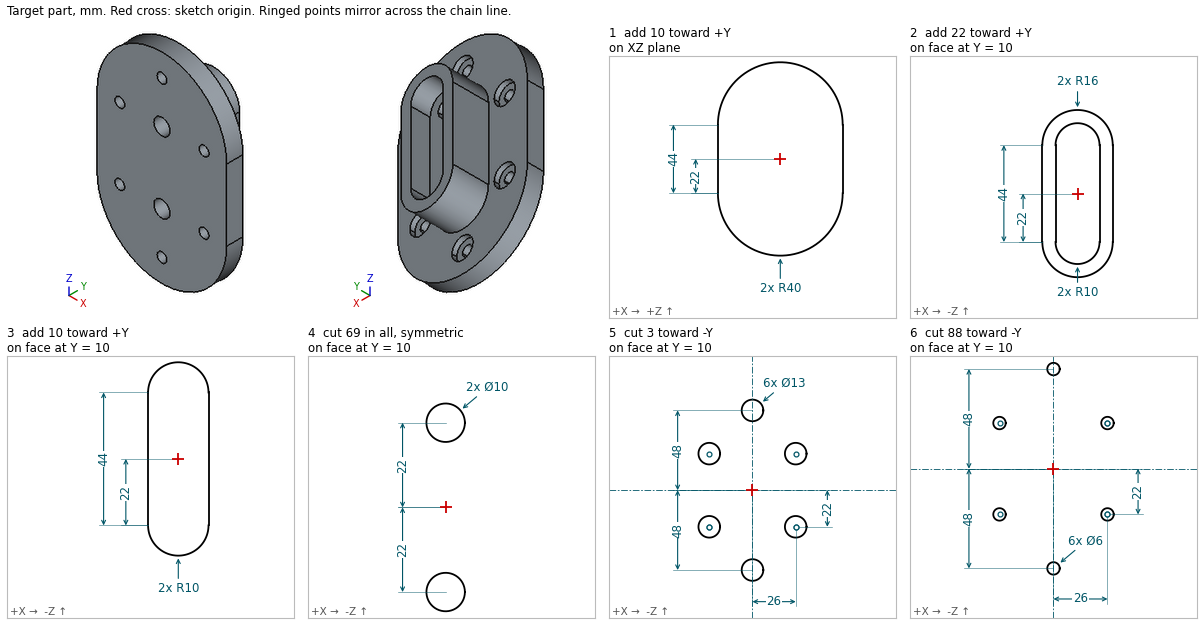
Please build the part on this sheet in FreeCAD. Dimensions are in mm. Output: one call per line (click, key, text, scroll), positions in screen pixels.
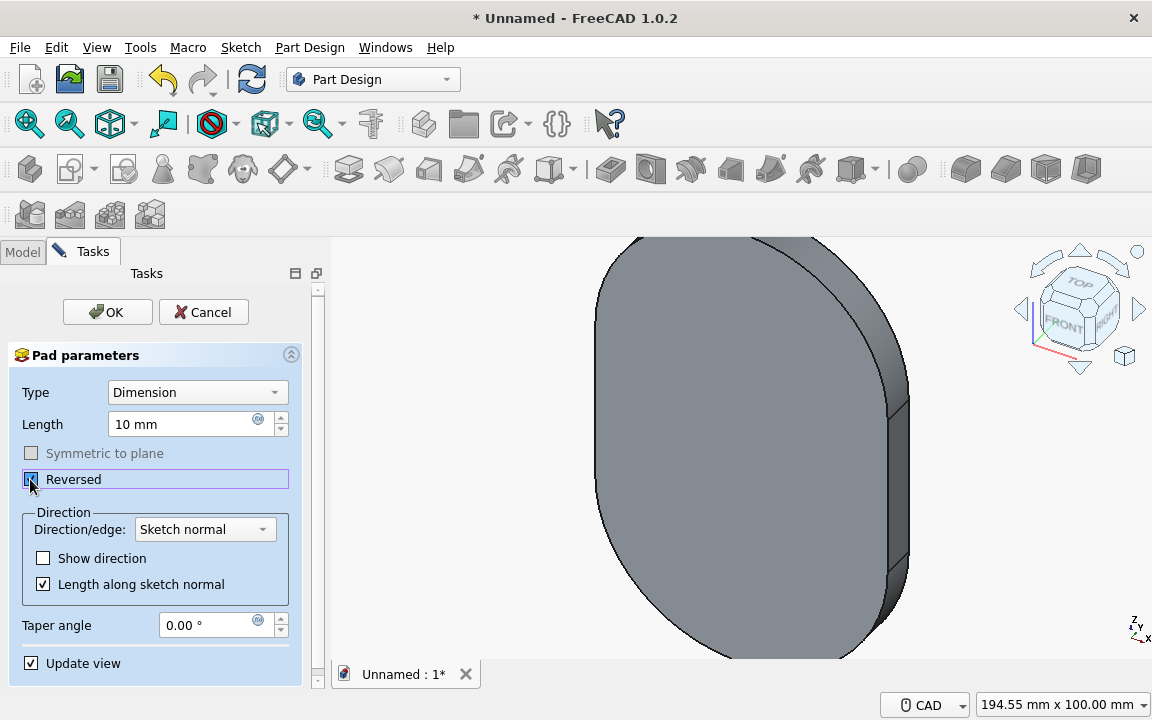
click(108, 312)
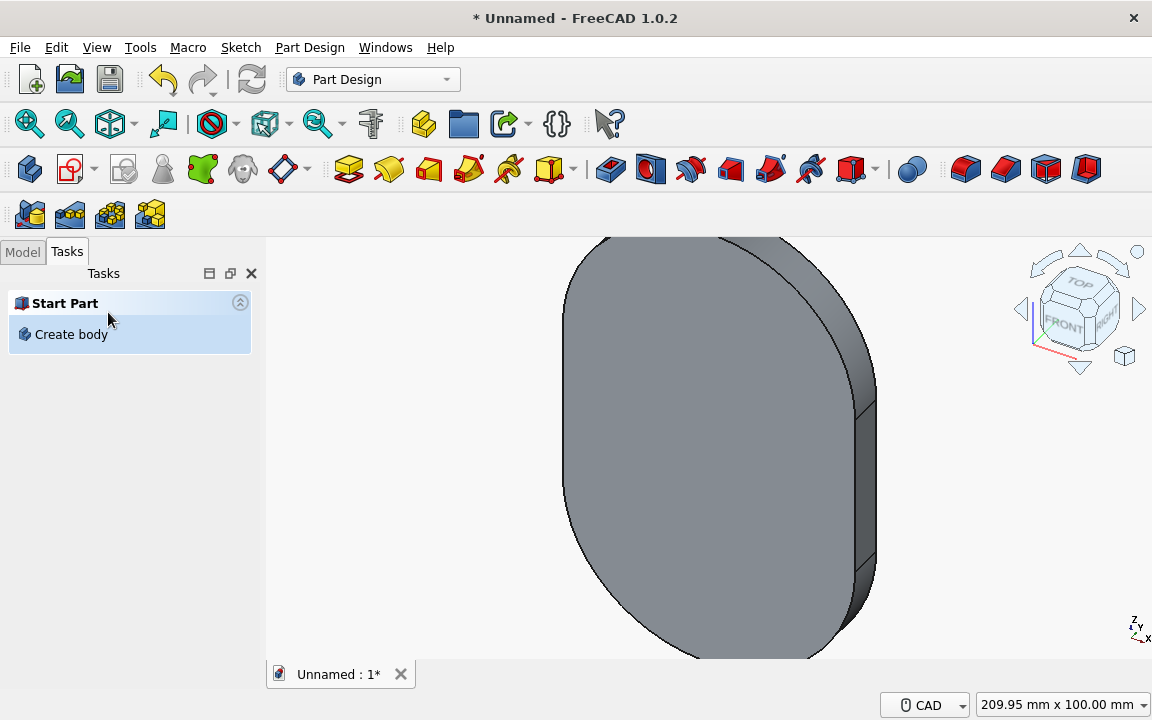
click(30, 124)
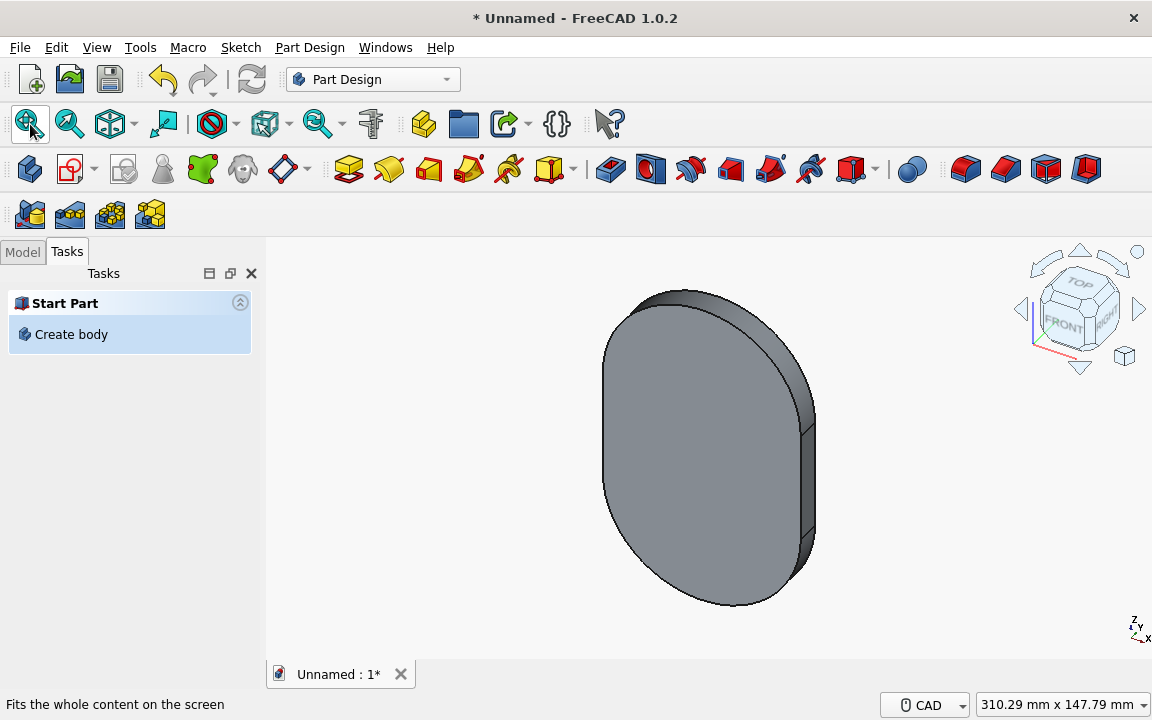
key(4)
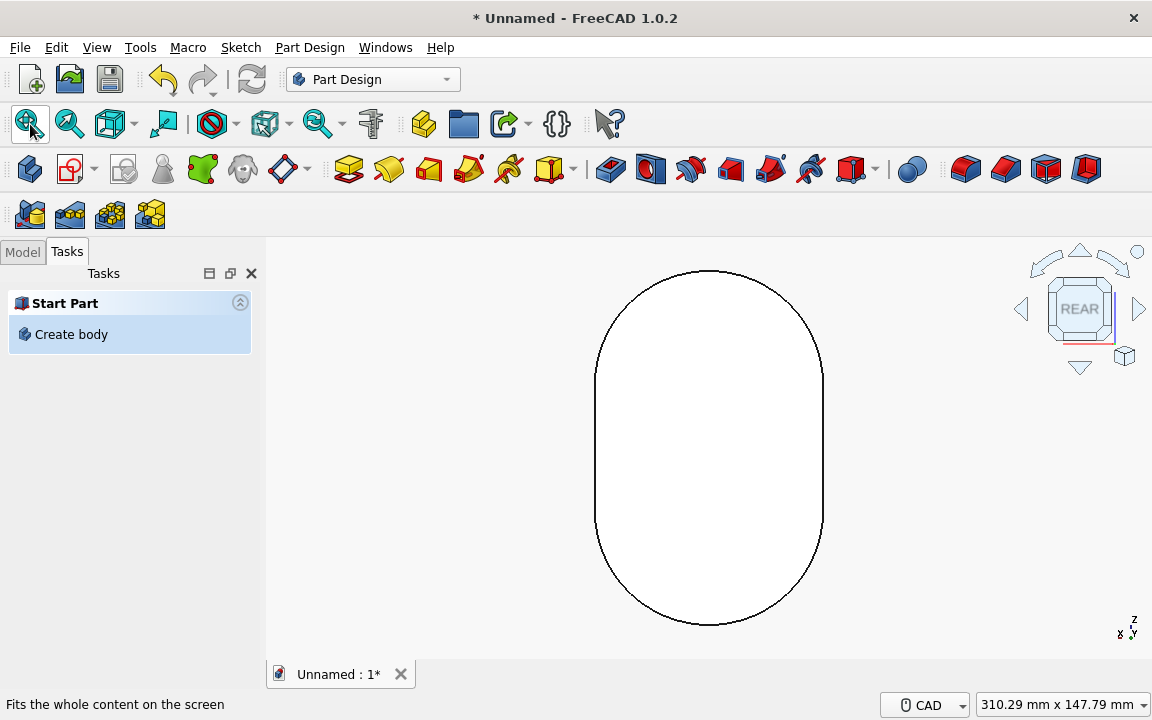
click(709, 396)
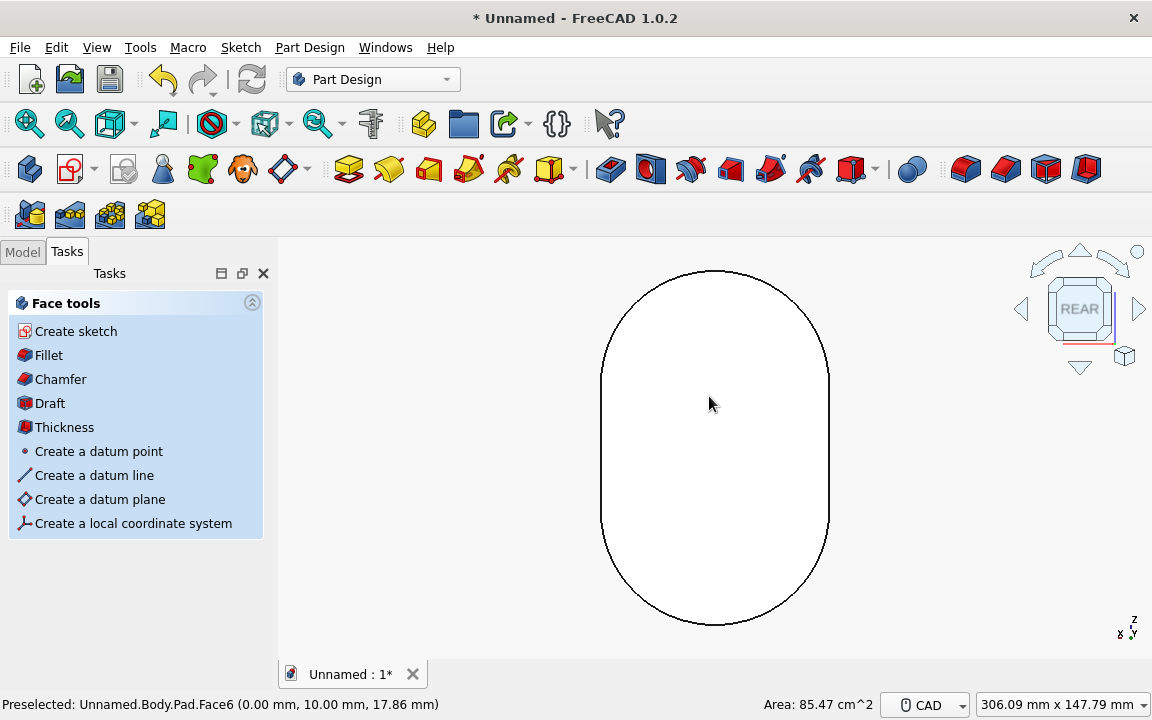
click(70, 170)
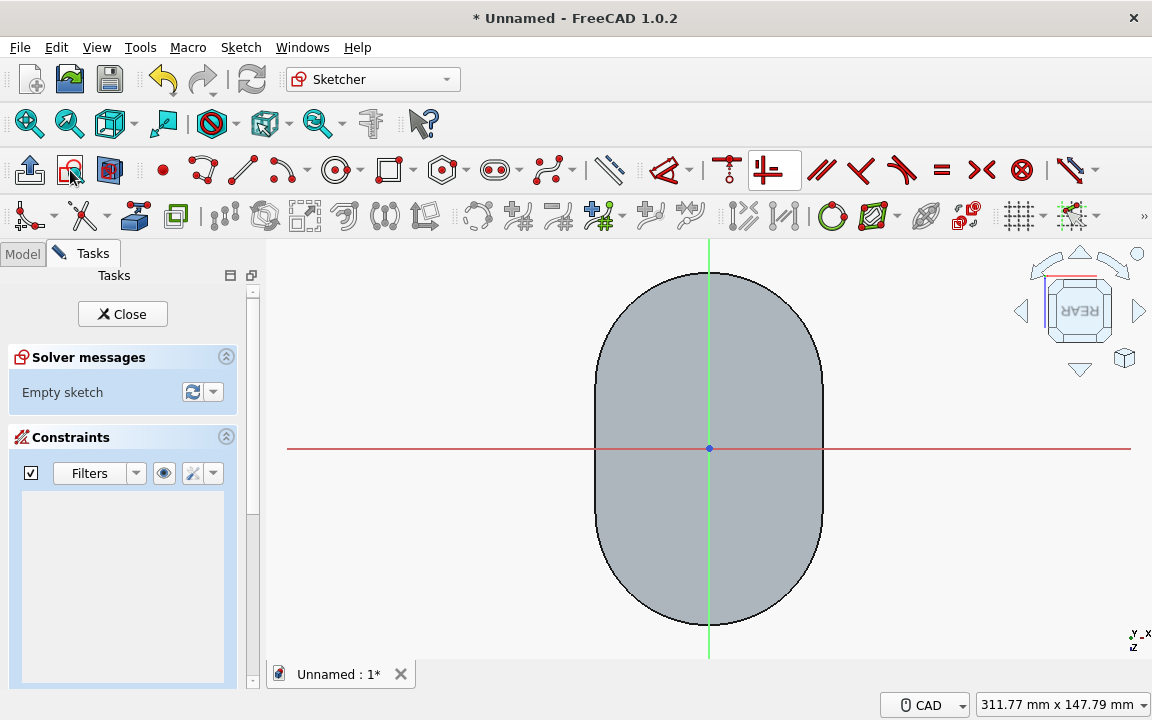
key(g)
key(s)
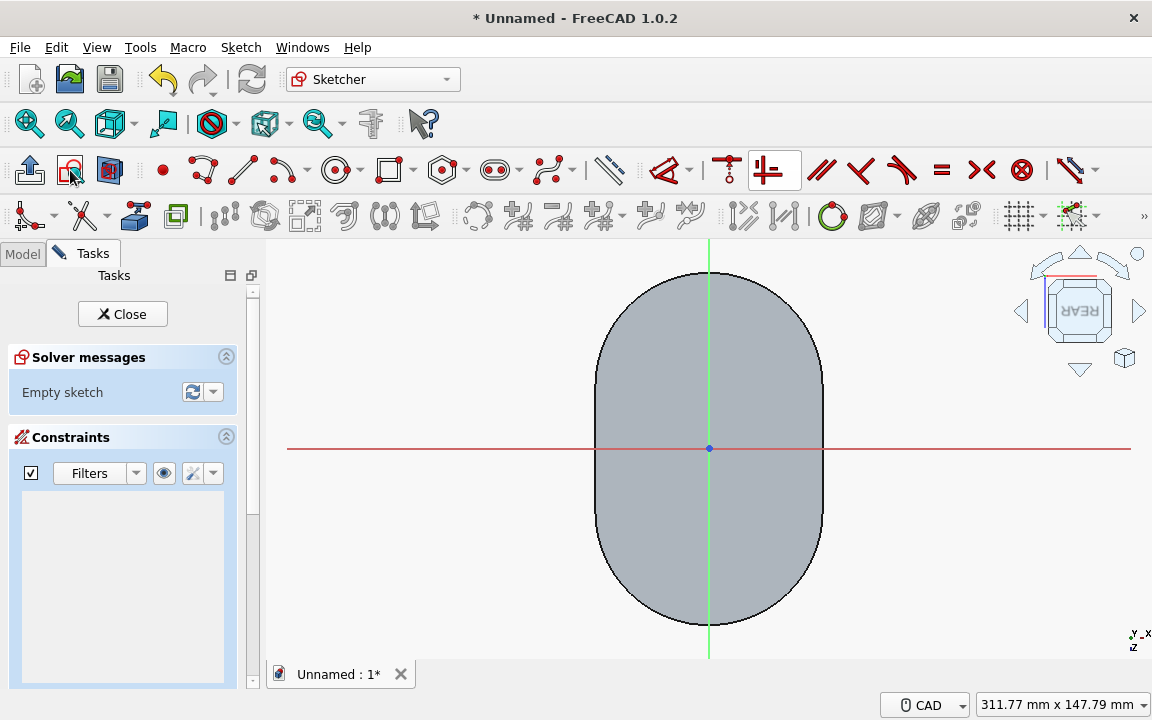
click(709, 512)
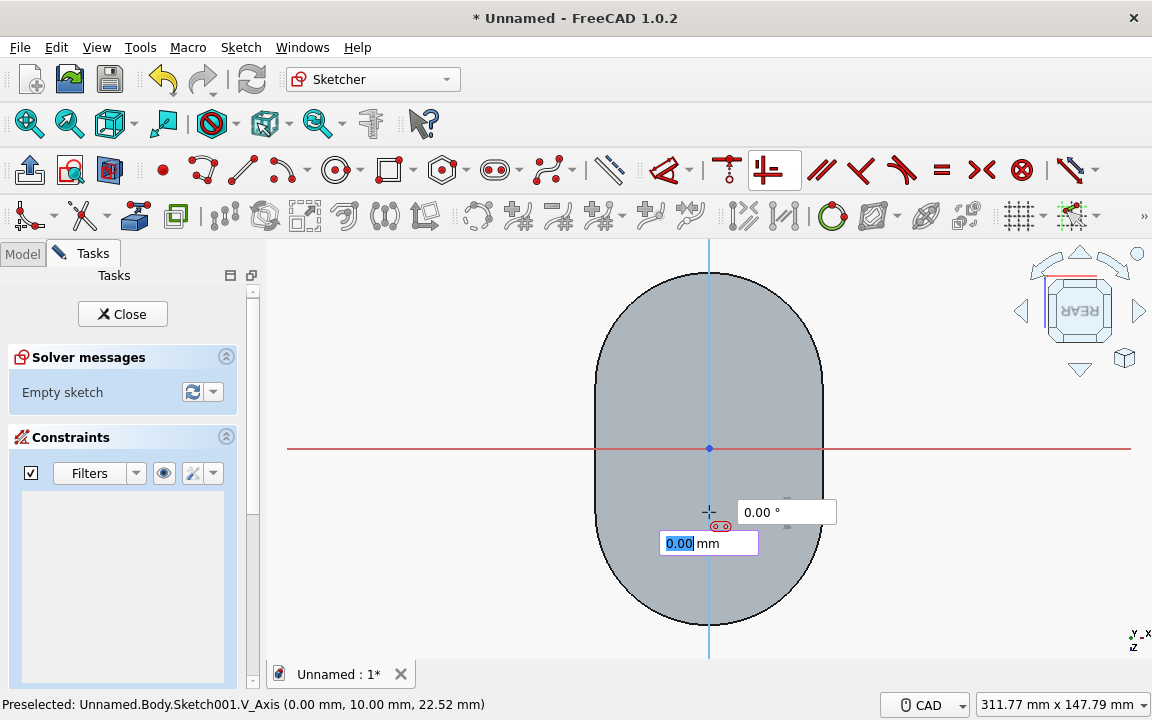
click(718, 386)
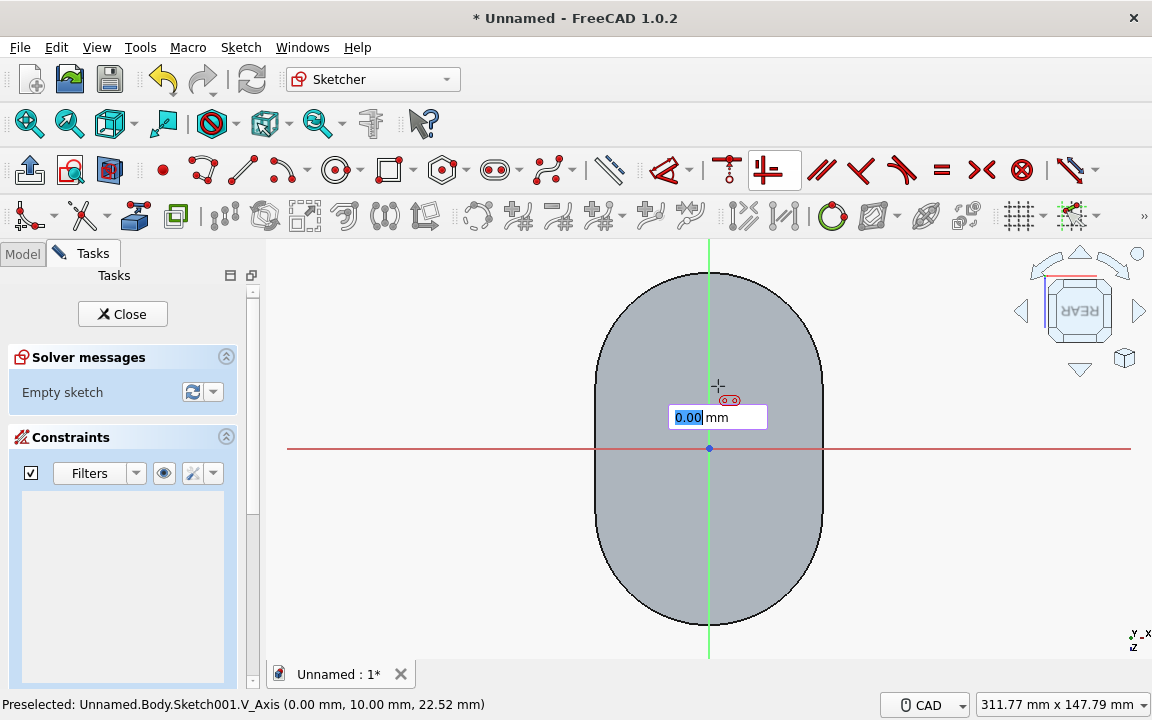
click(754, 468)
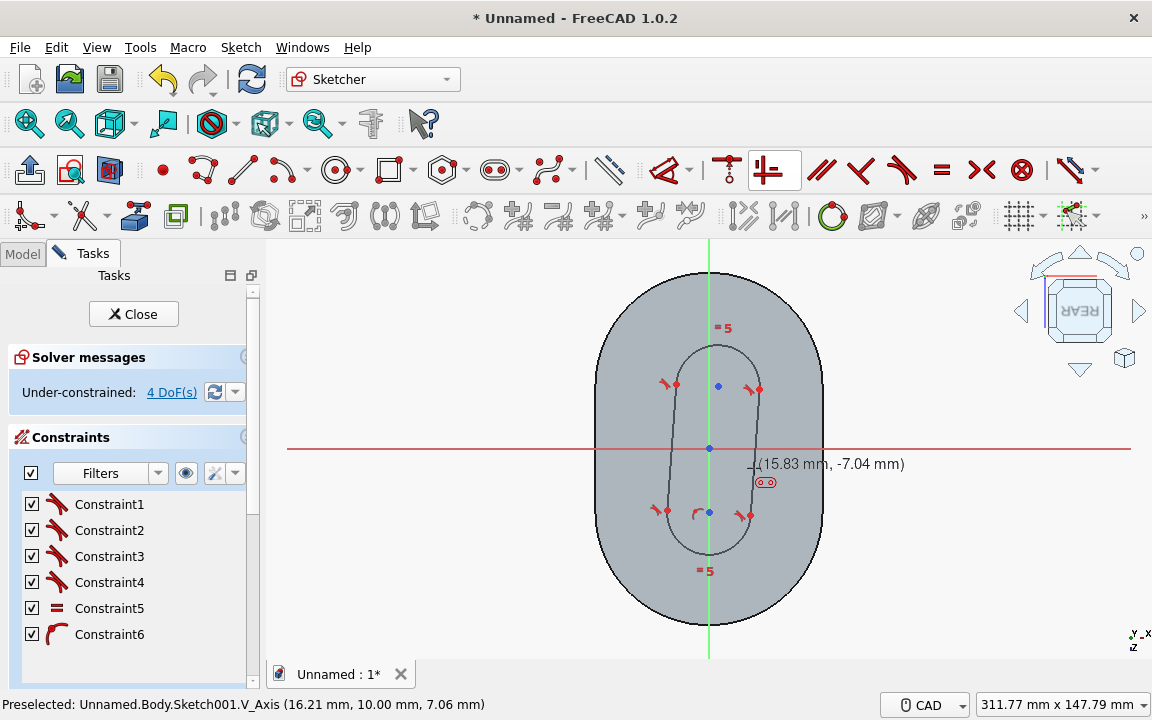
click(709, 513)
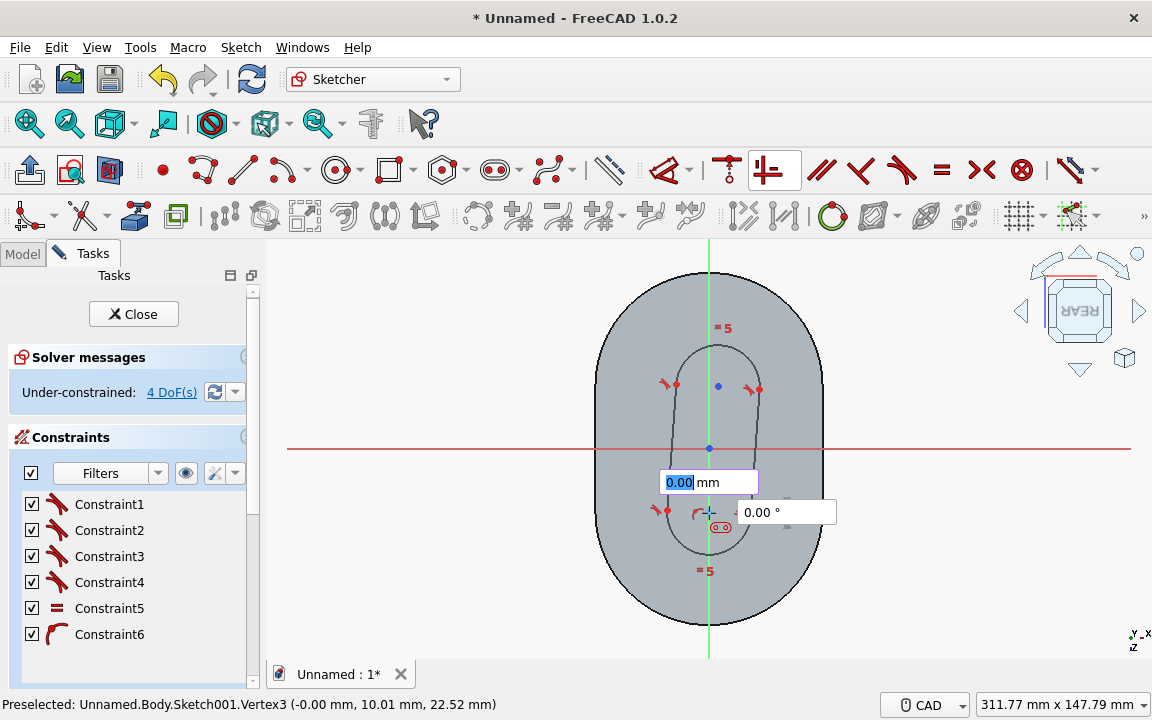
click(718, 387)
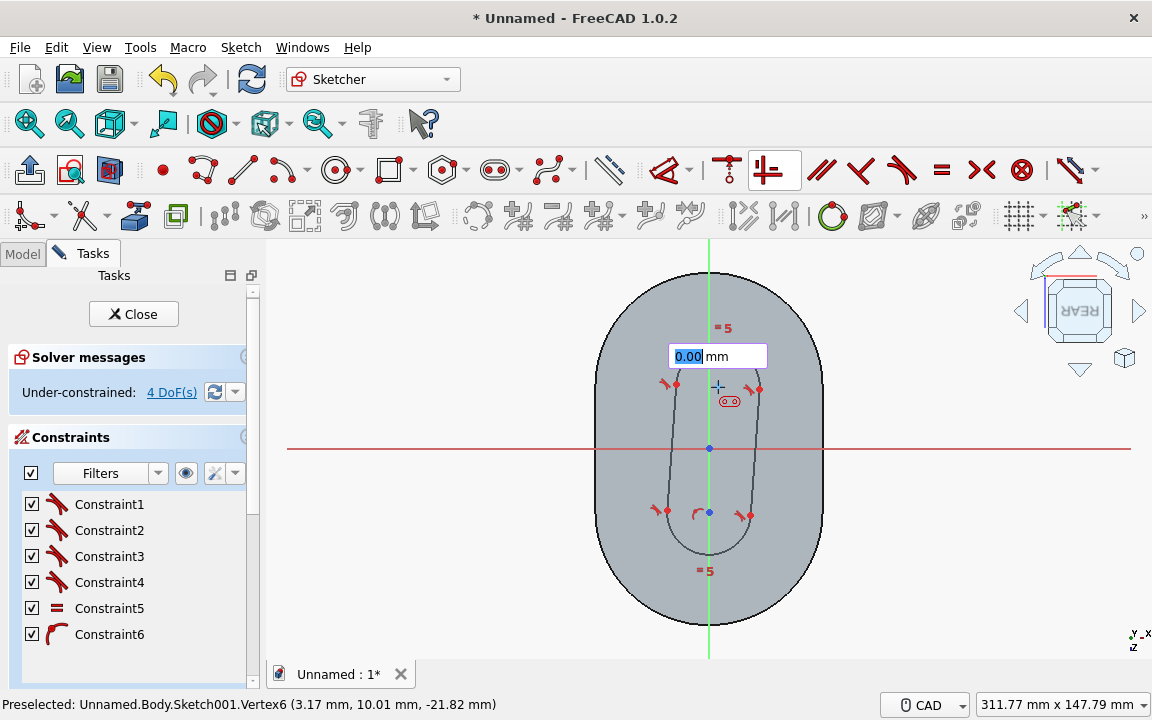
click(737, 430)
key(Escape)